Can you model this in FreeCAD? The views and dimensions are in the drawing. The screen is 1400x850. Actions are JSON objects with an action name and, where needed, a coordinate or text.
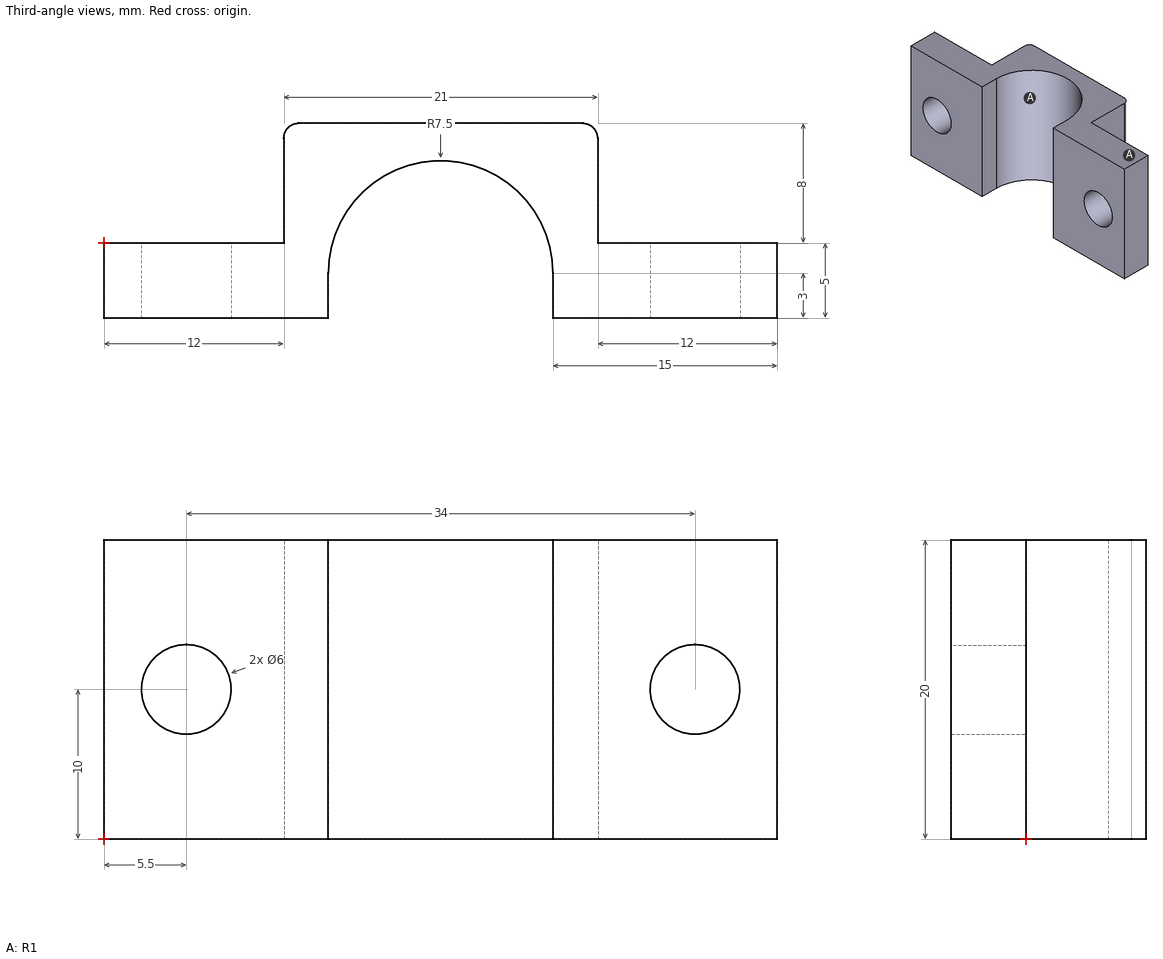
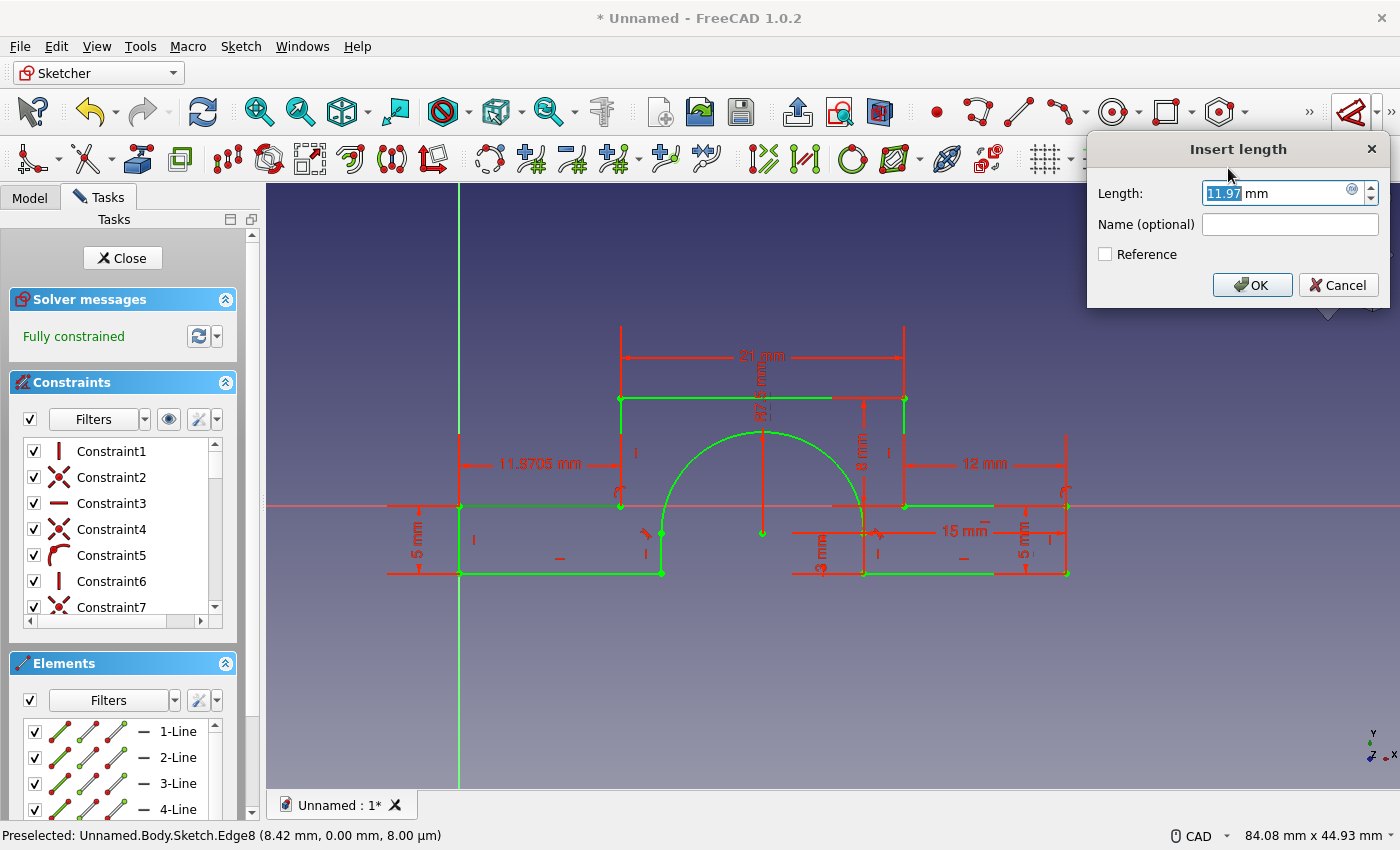
{"action": "type", "text": "12"}
{"action": "key", "text": "Return"}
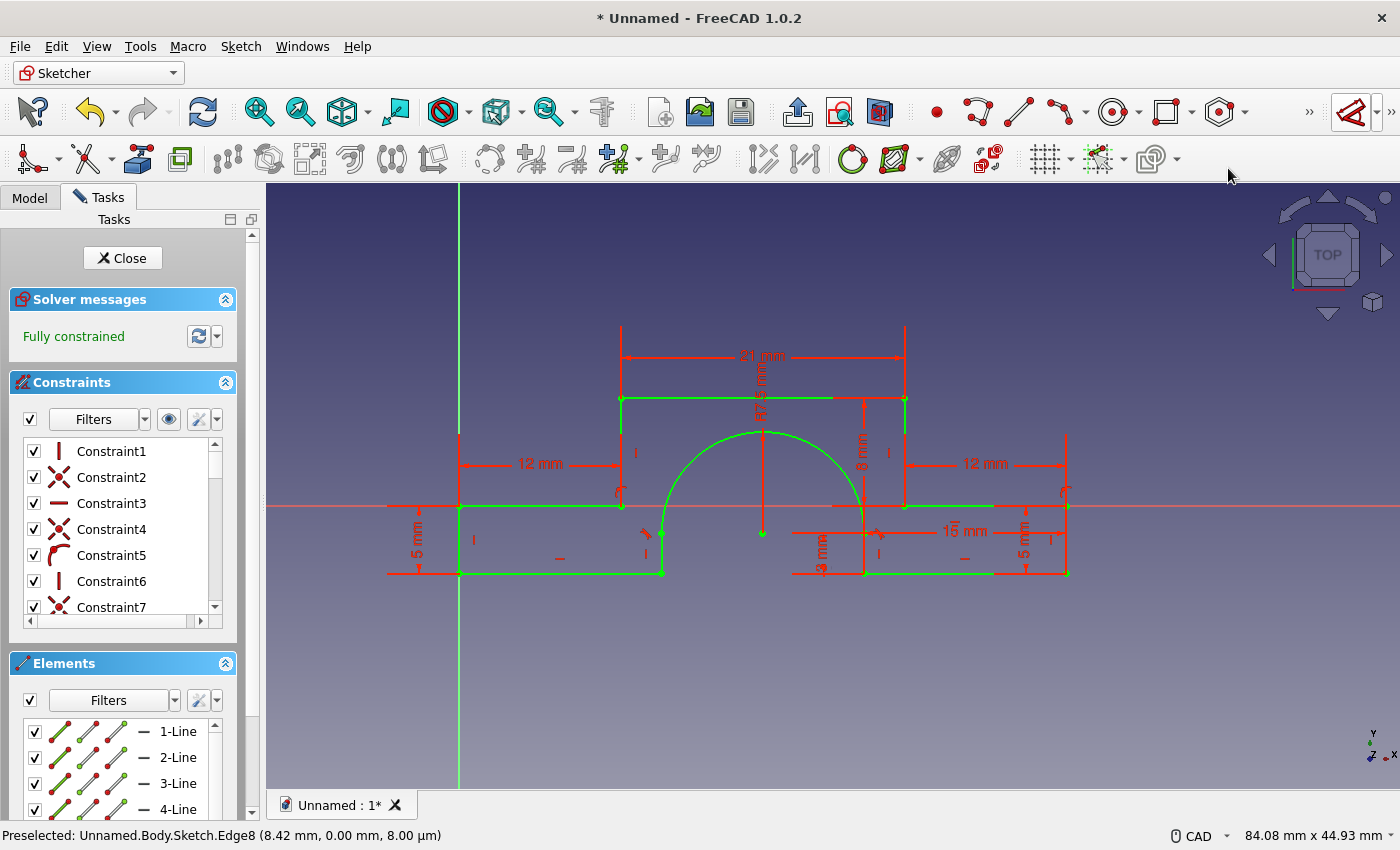
{"action": "left_click", "coordinate": [123, 258]}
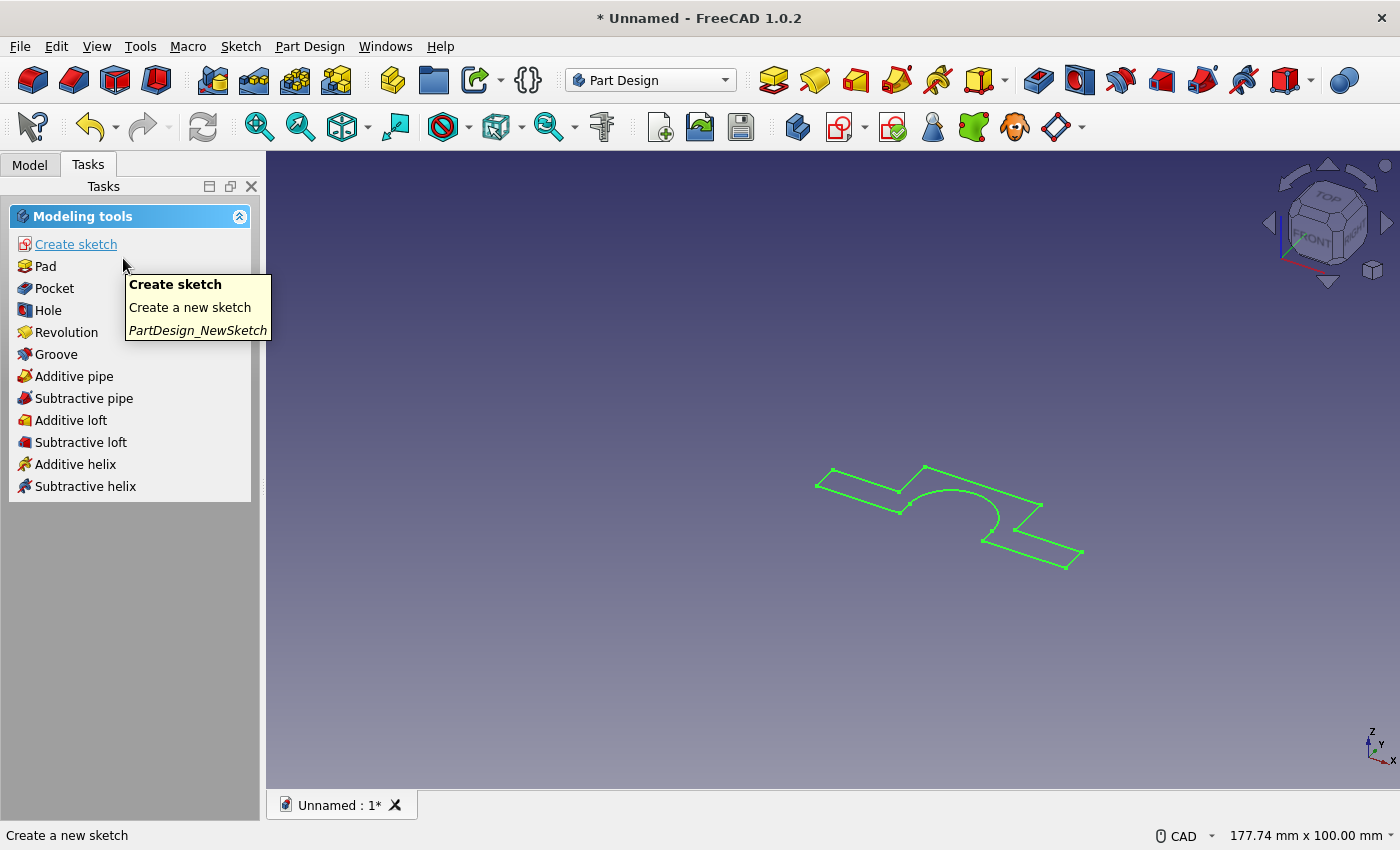
{"action": "left_click", "coordinate": [774, 80]}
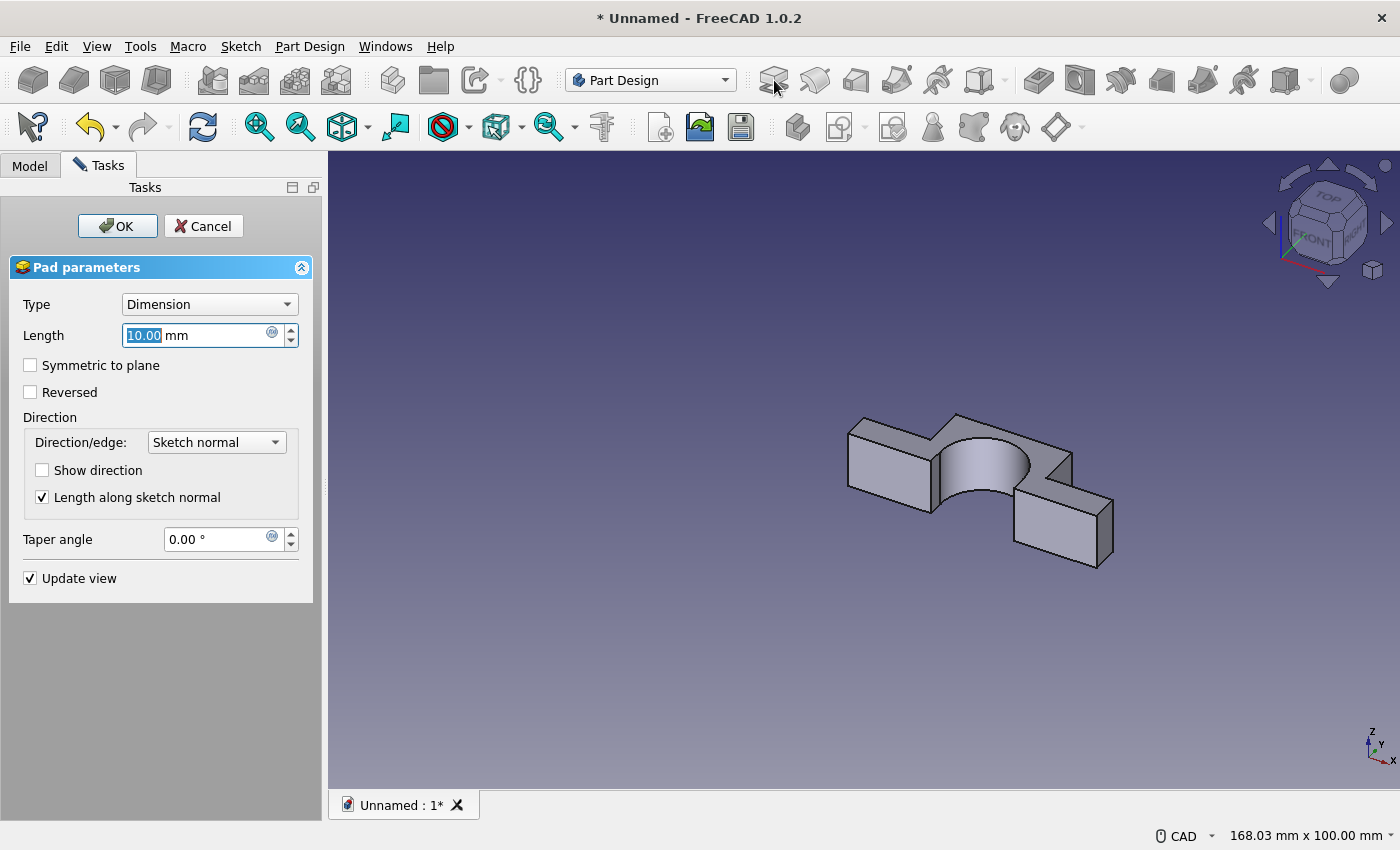
{"action": "type", "text": "20"}
{"action": "key", "text": "Tab"}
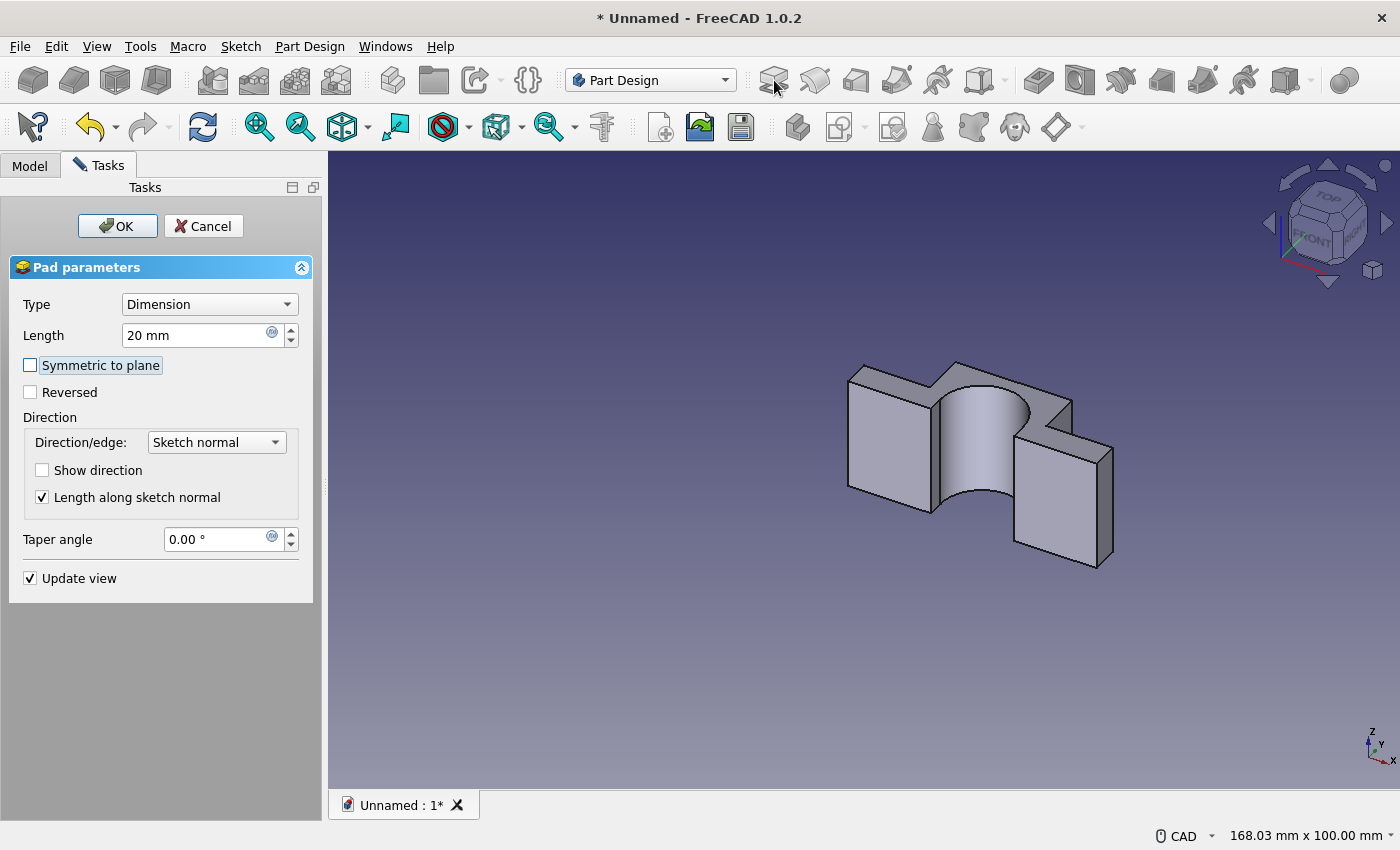
{"action": "left_click", "coordinate": [118, 226]}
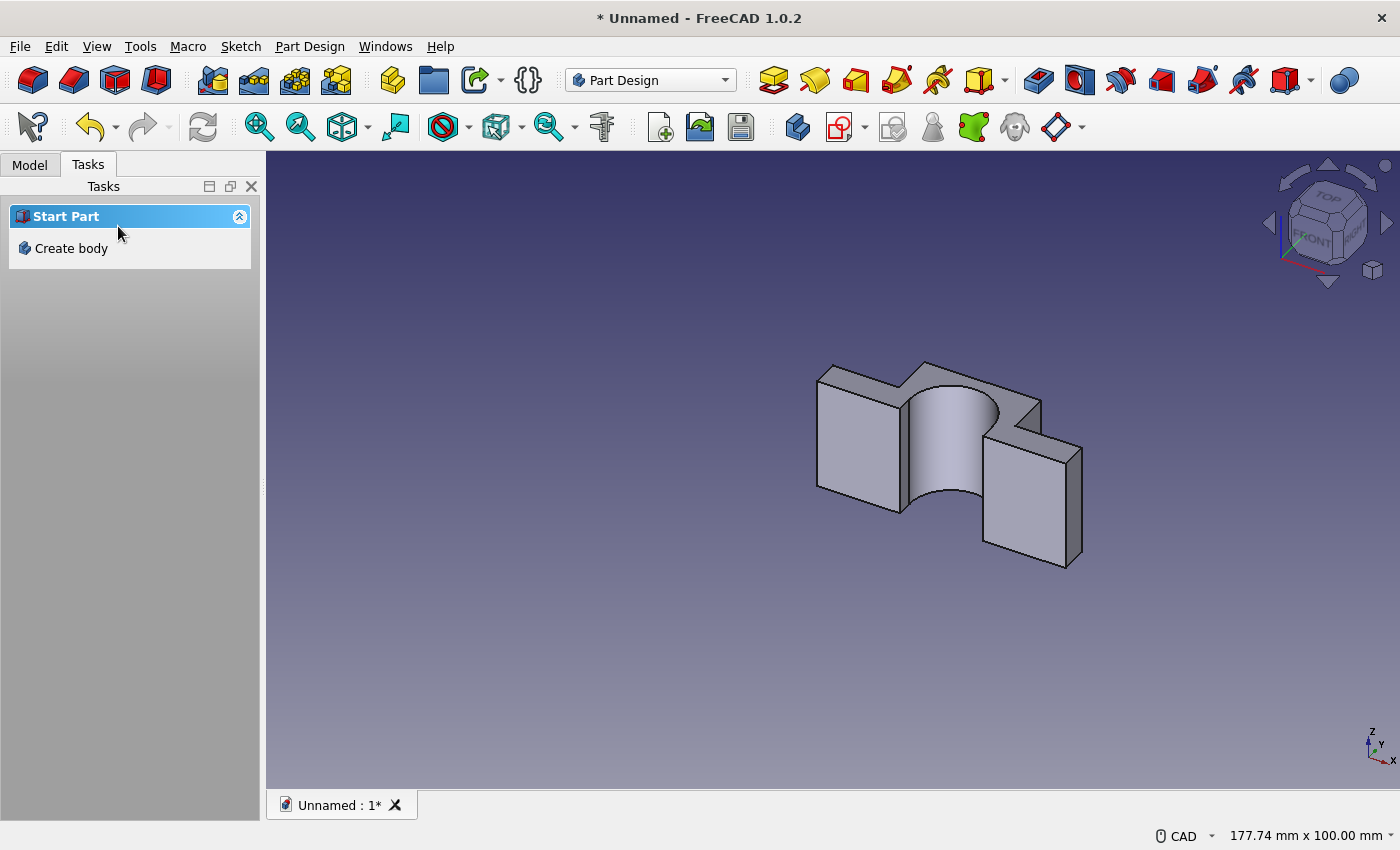
{"action": "left_click", "coordinate": [260, 128]}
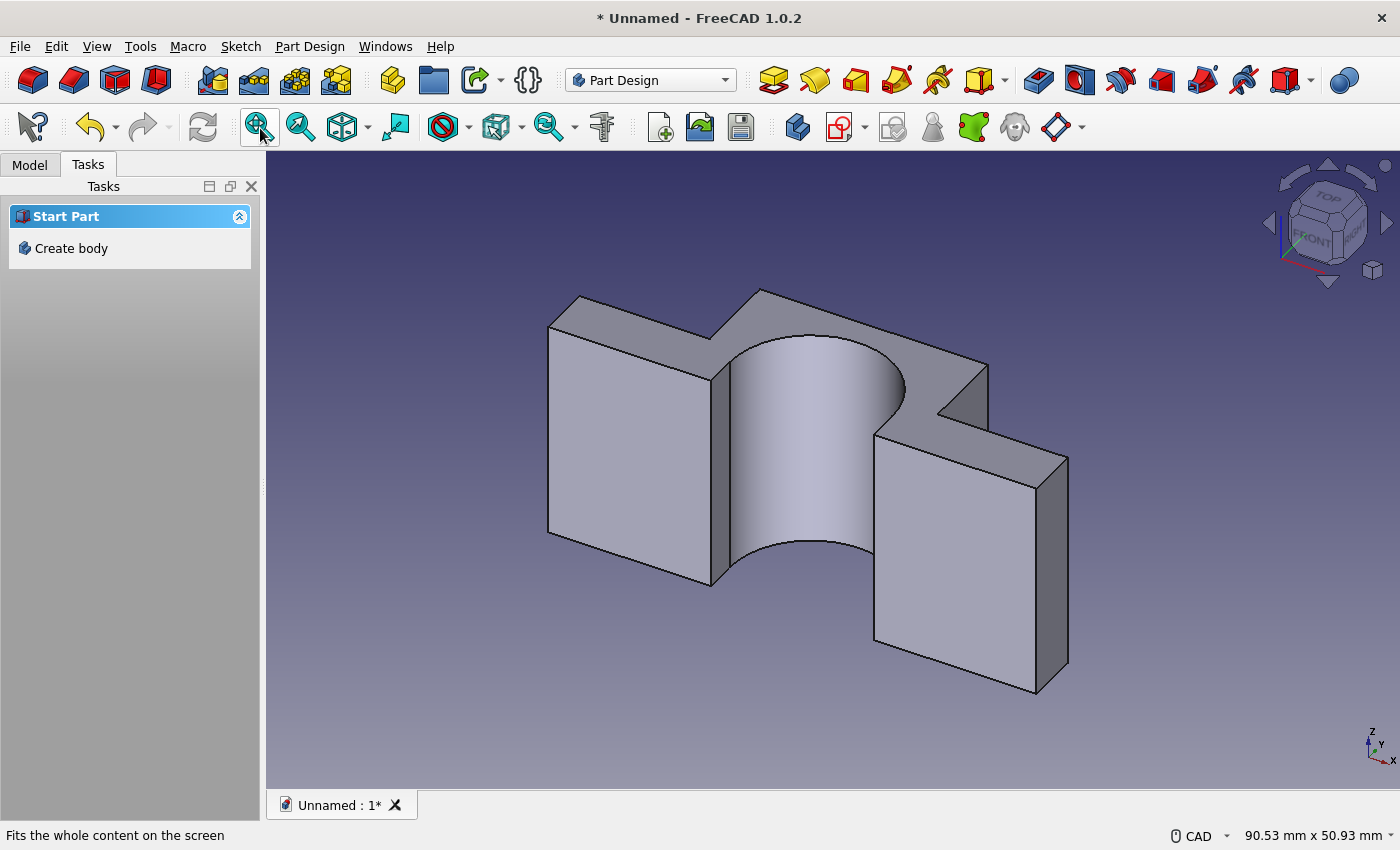
{"action": "key", "text": "0"}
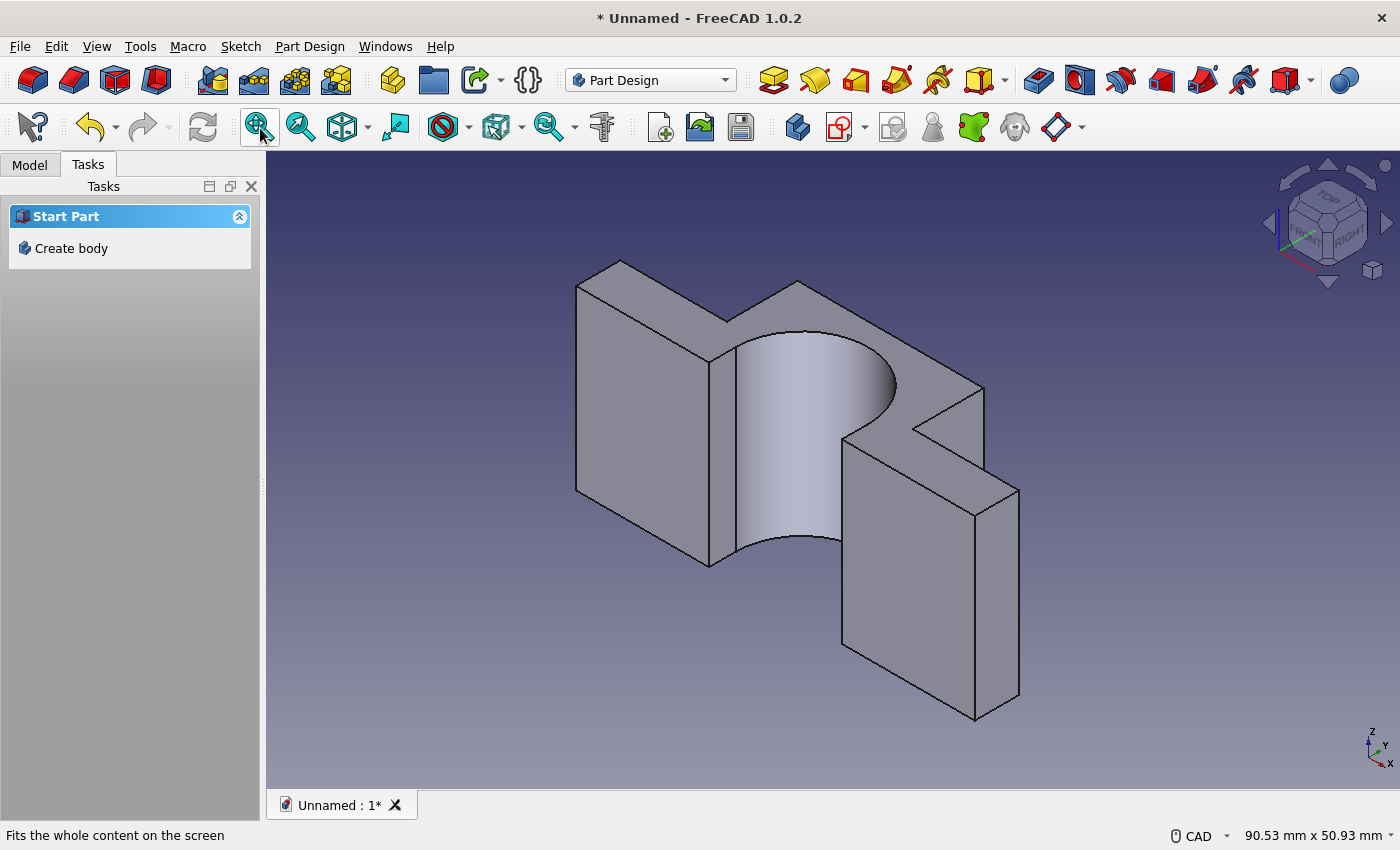
{"action": "key", "text": "2"}